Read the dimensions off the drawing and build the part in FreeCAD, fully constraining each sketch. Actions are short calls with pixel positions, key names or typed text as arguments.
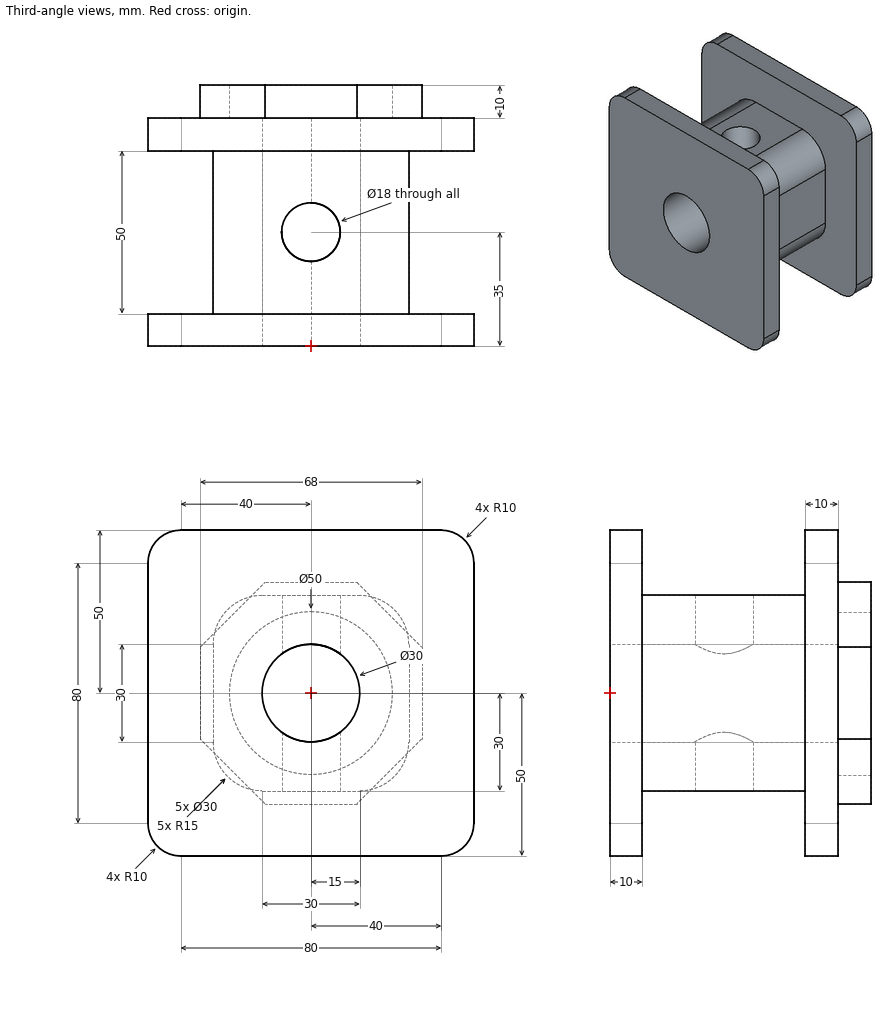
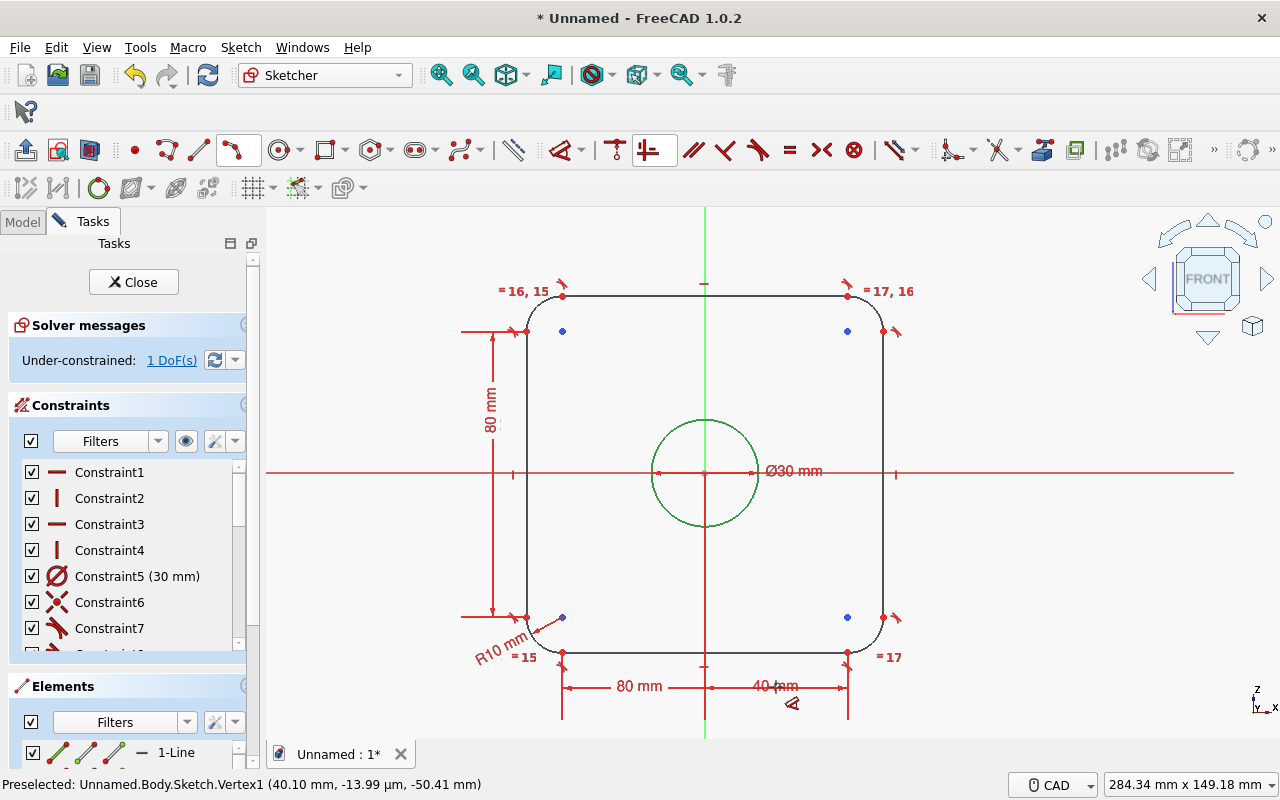
click(848, 653)
click(671, 563)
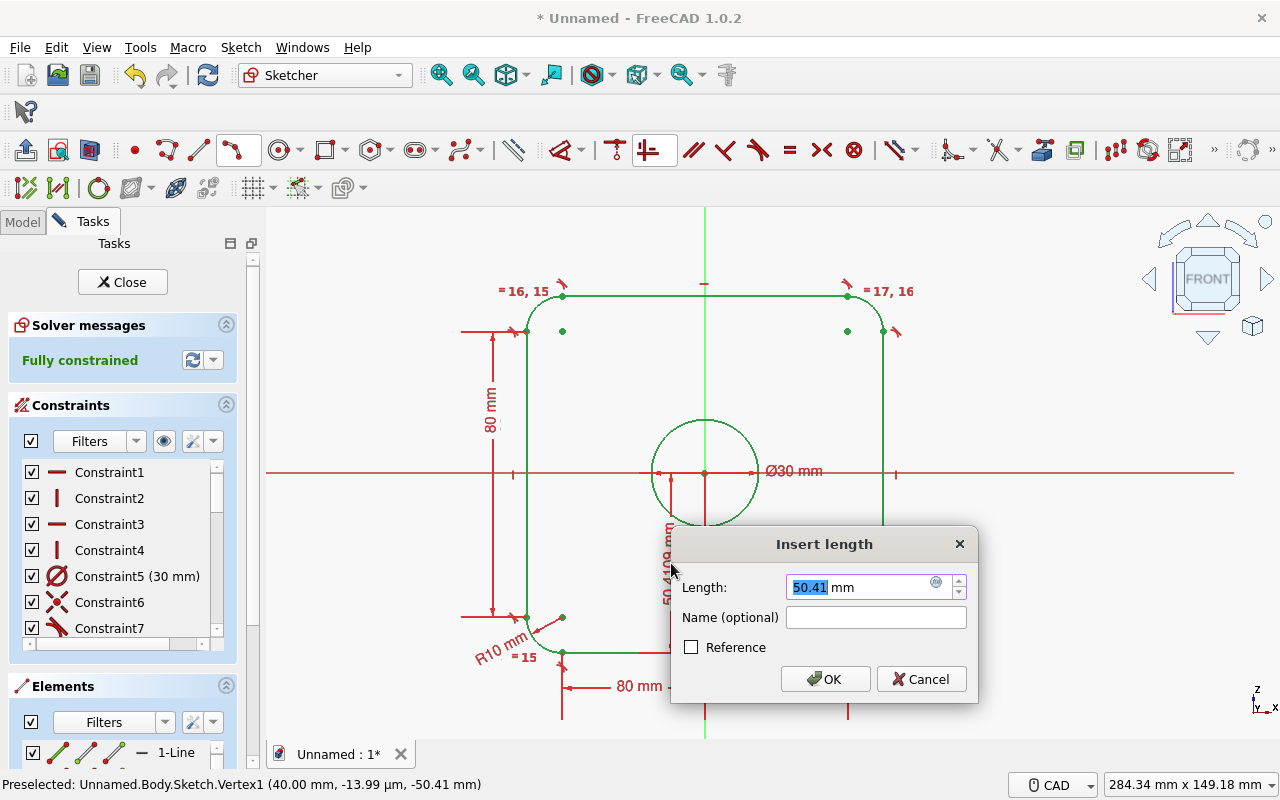
text(50)
key(Return)
key(Escape)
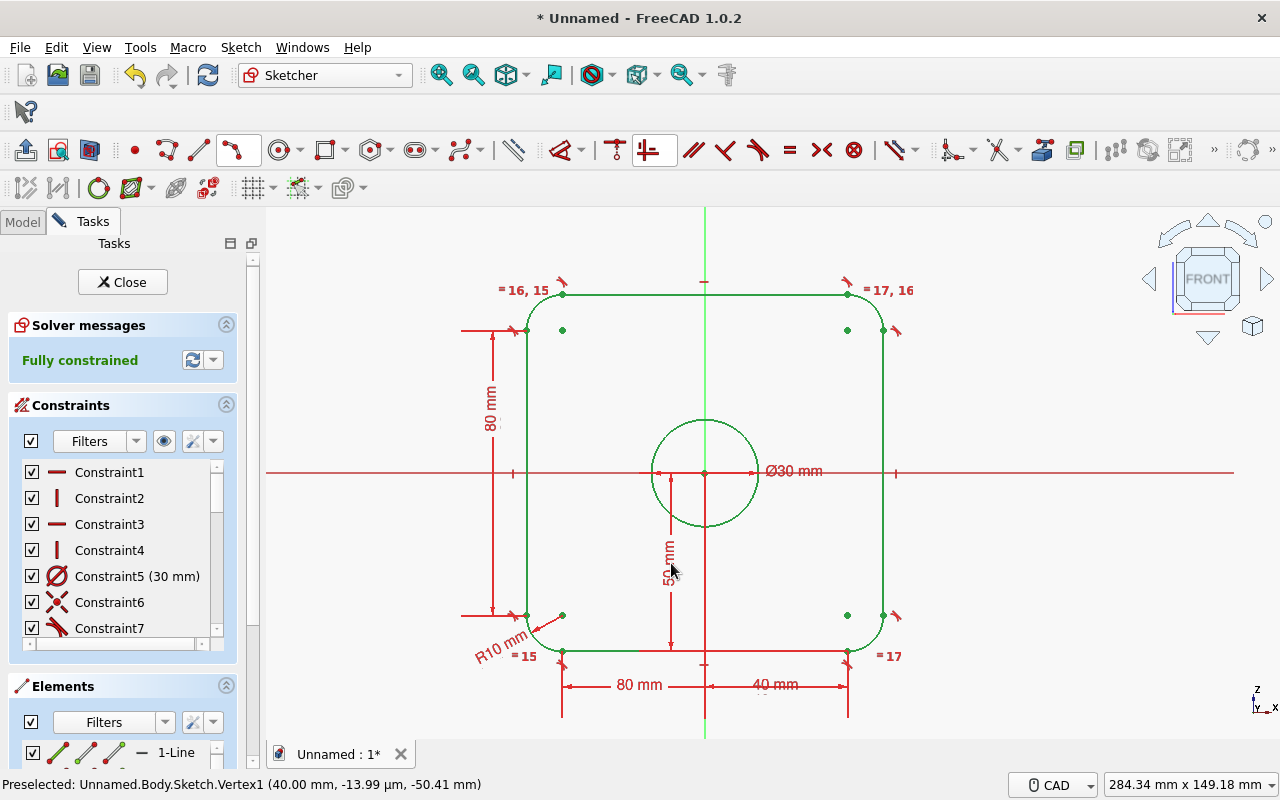
click(123, 282)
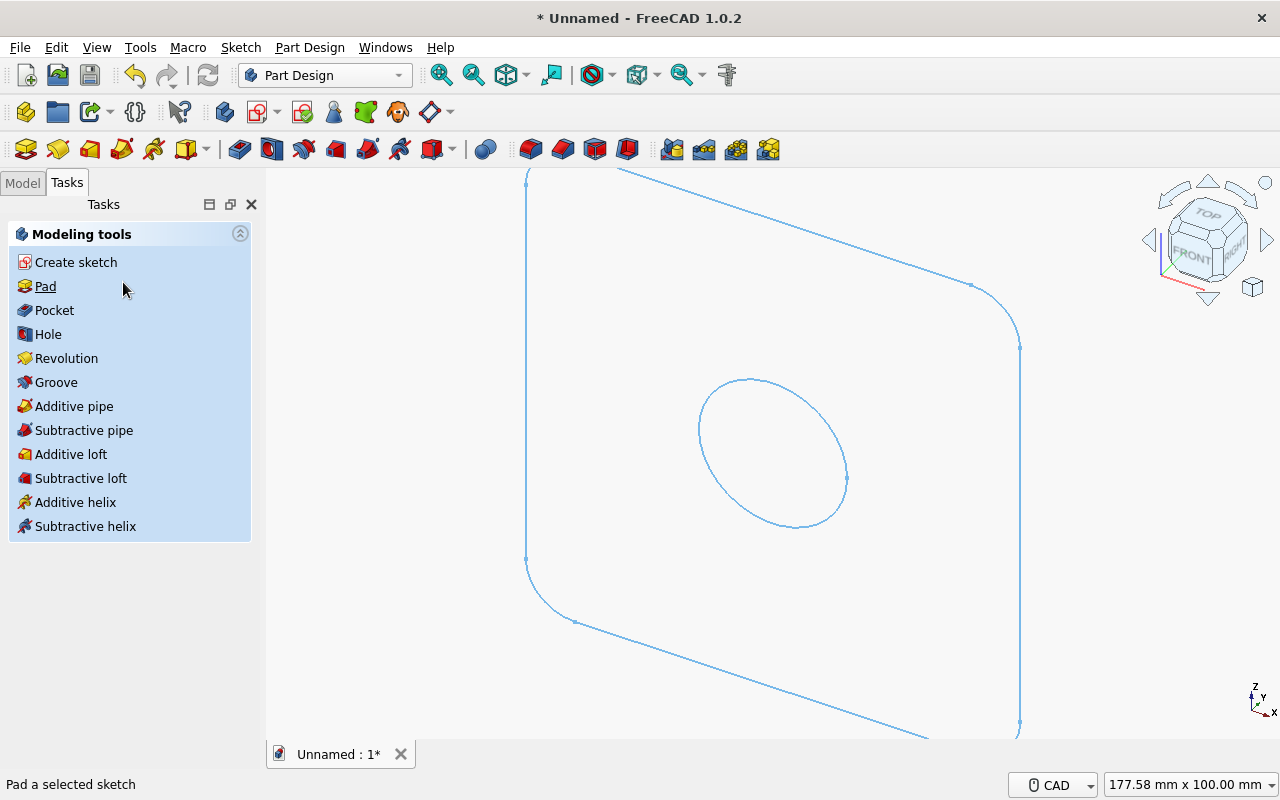
click(26, 150)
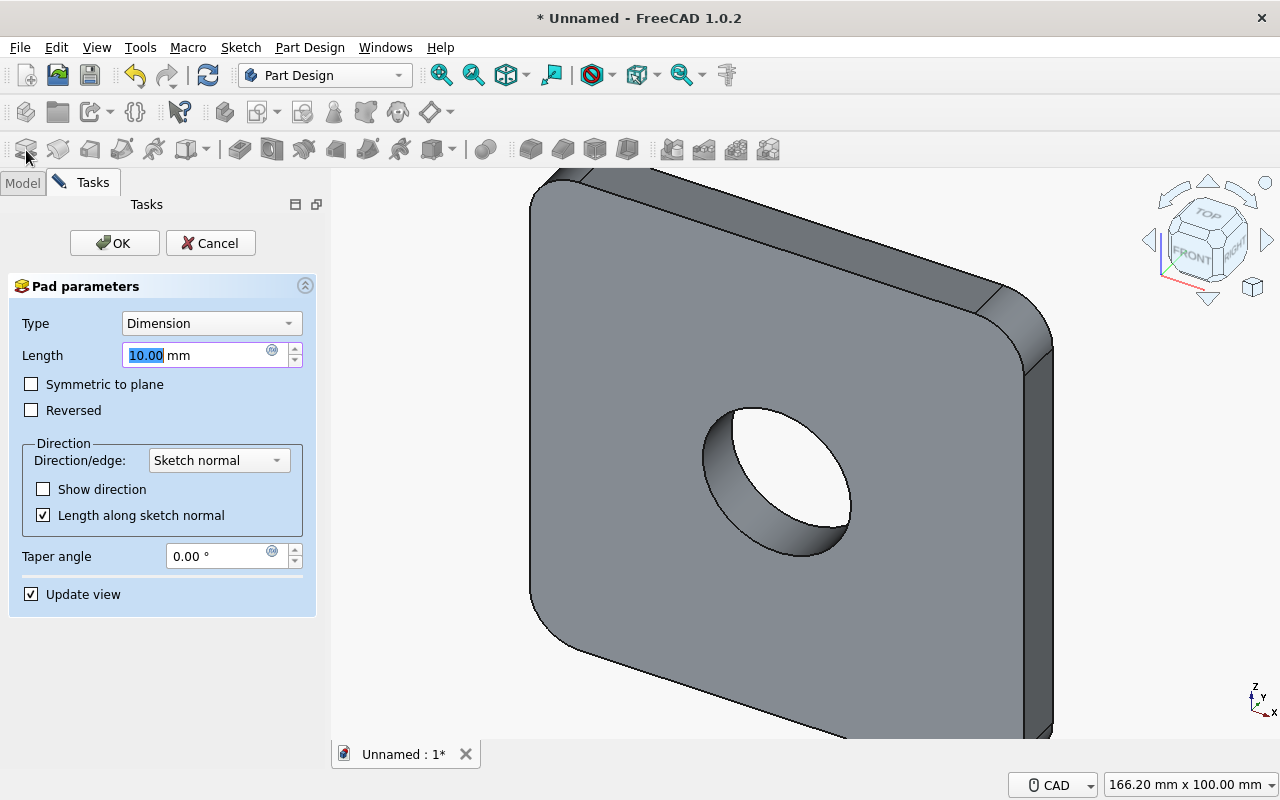
text(10)
key(Tab)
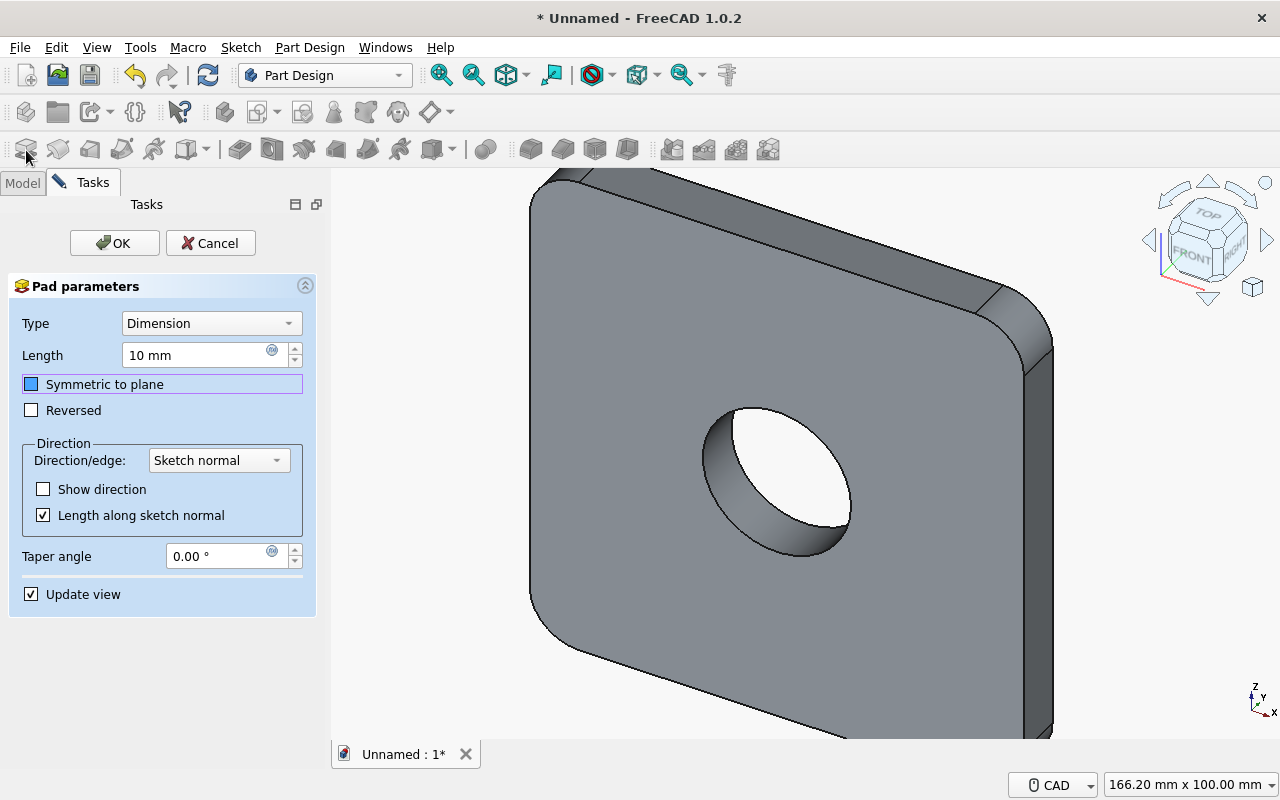
click(30, 410)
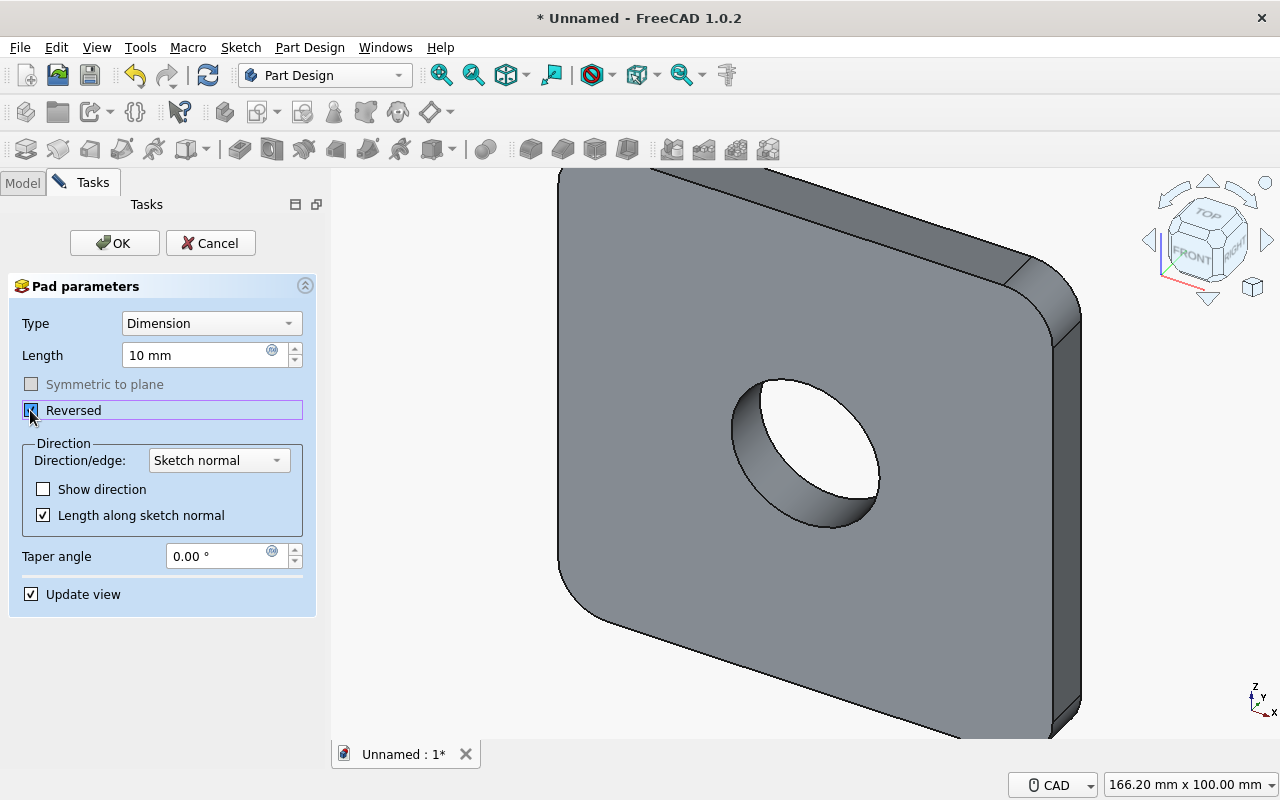
click(115, 243)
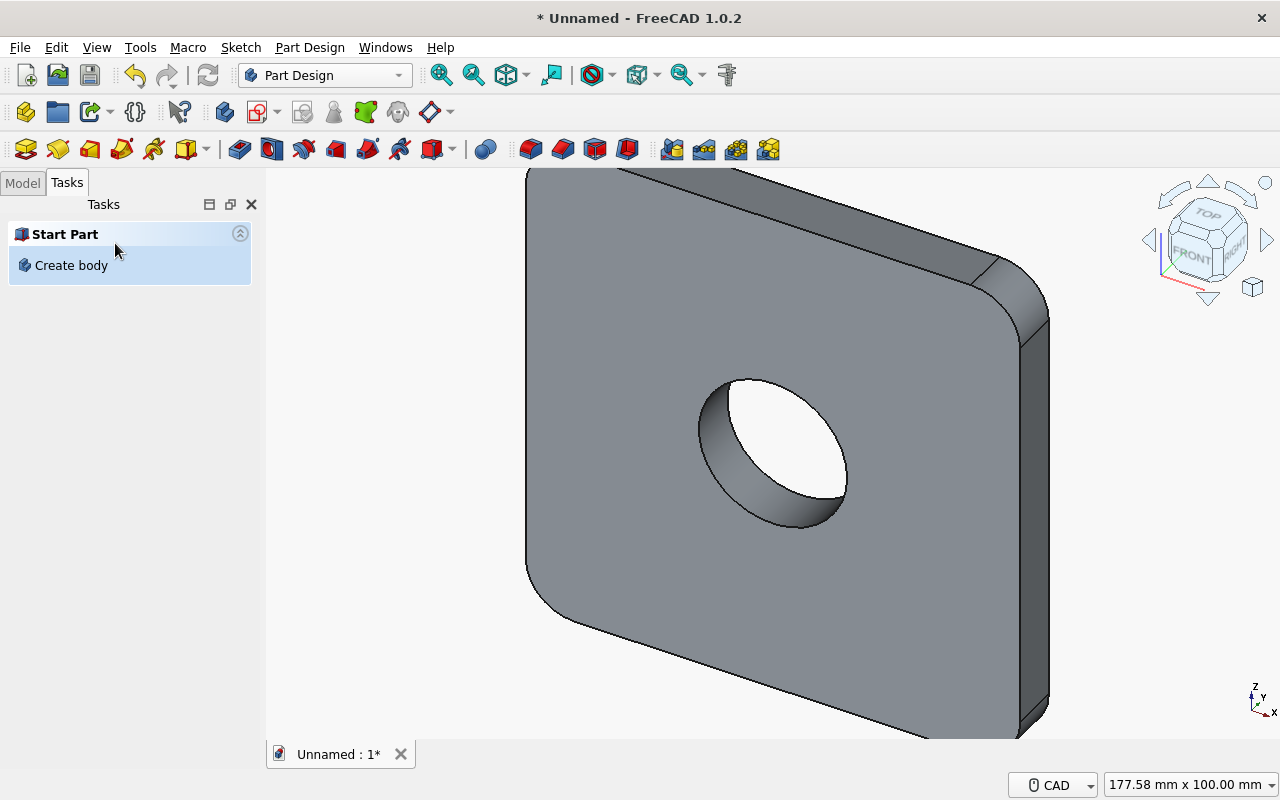
click(442, 76)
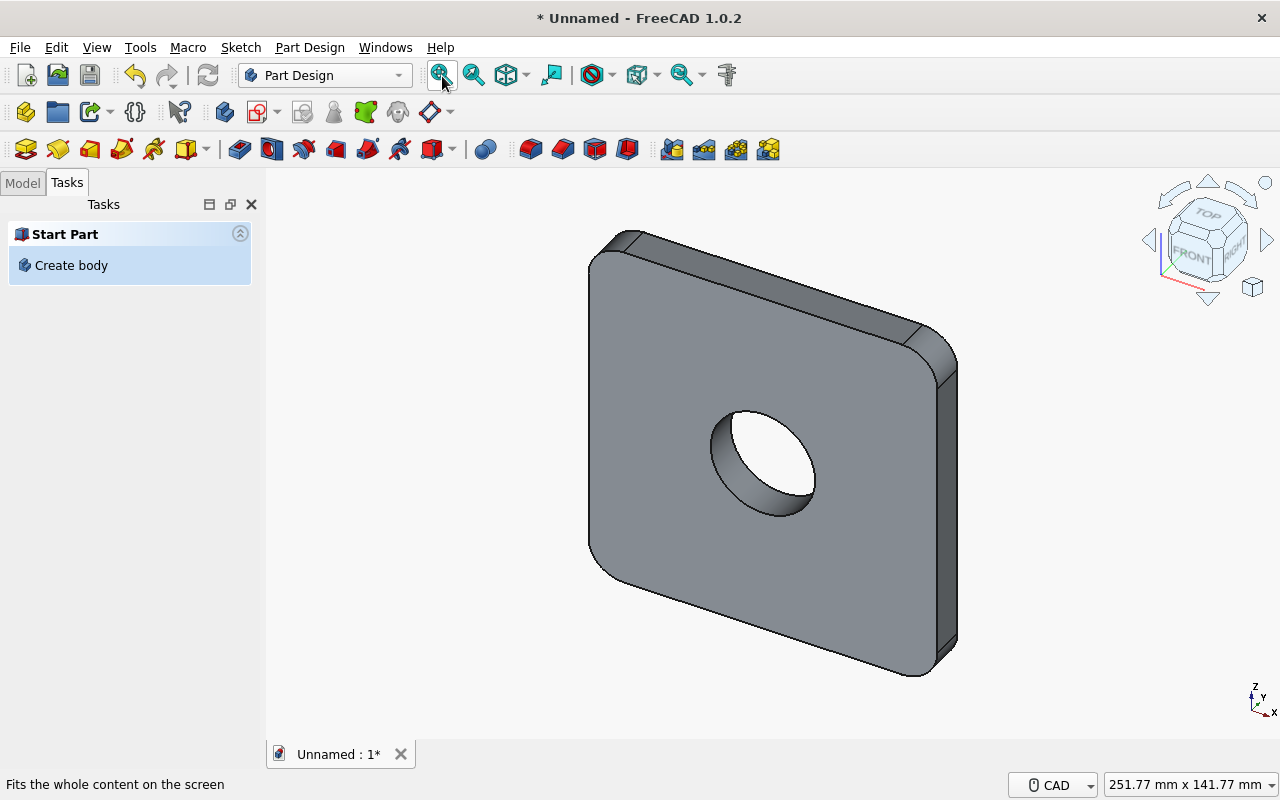
key(4)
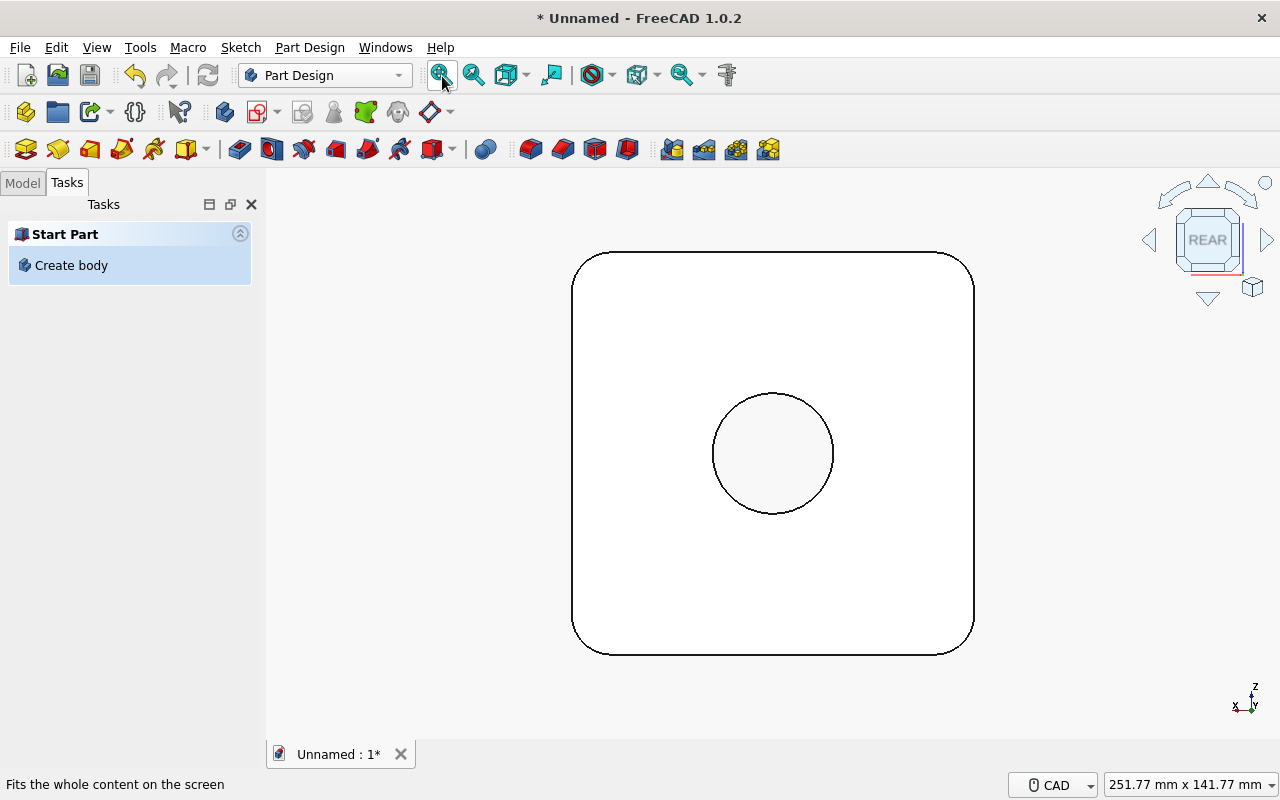
click(888, 337)